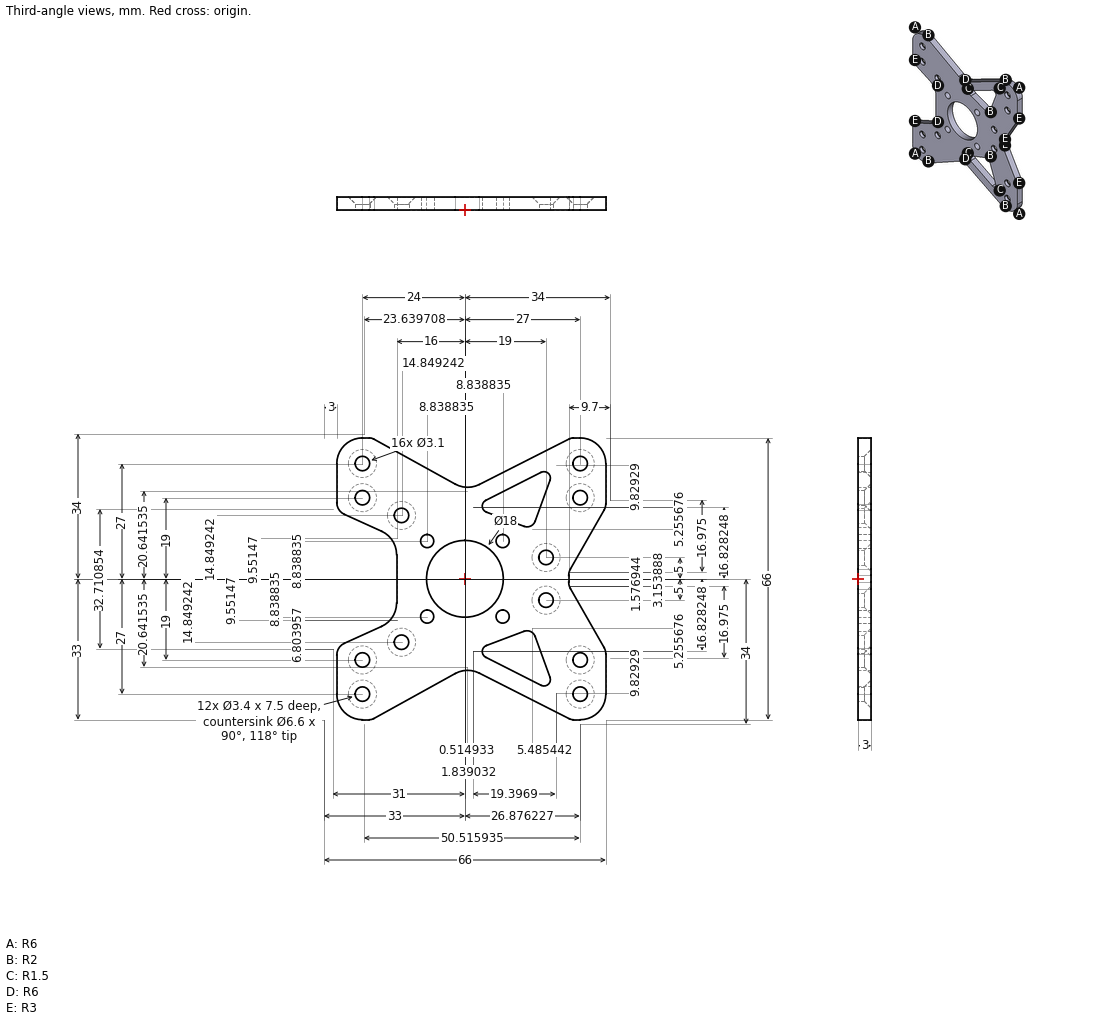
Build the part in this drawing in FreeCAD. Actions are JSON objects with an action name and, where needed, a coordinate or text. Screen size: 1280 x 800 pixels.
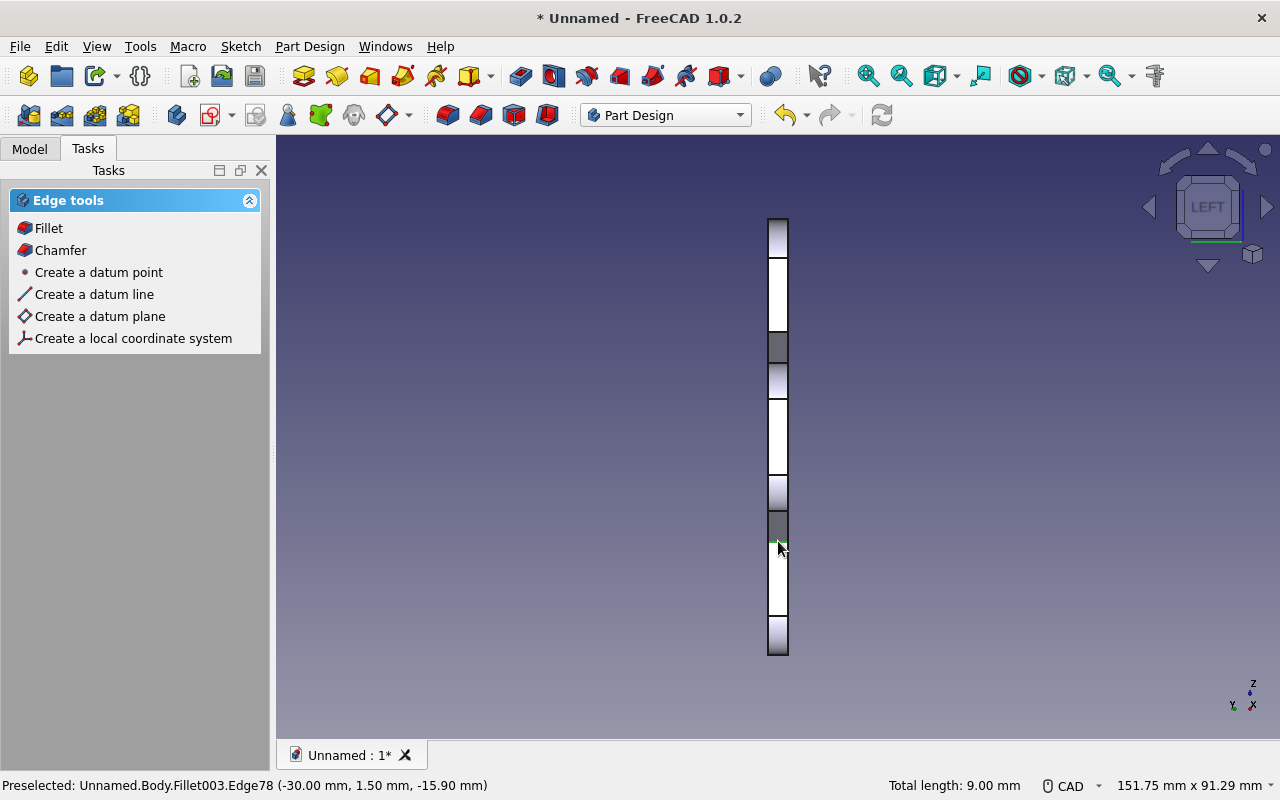
{"action": "left_click", "coordinate": [778, 331], "text": "ctrl"}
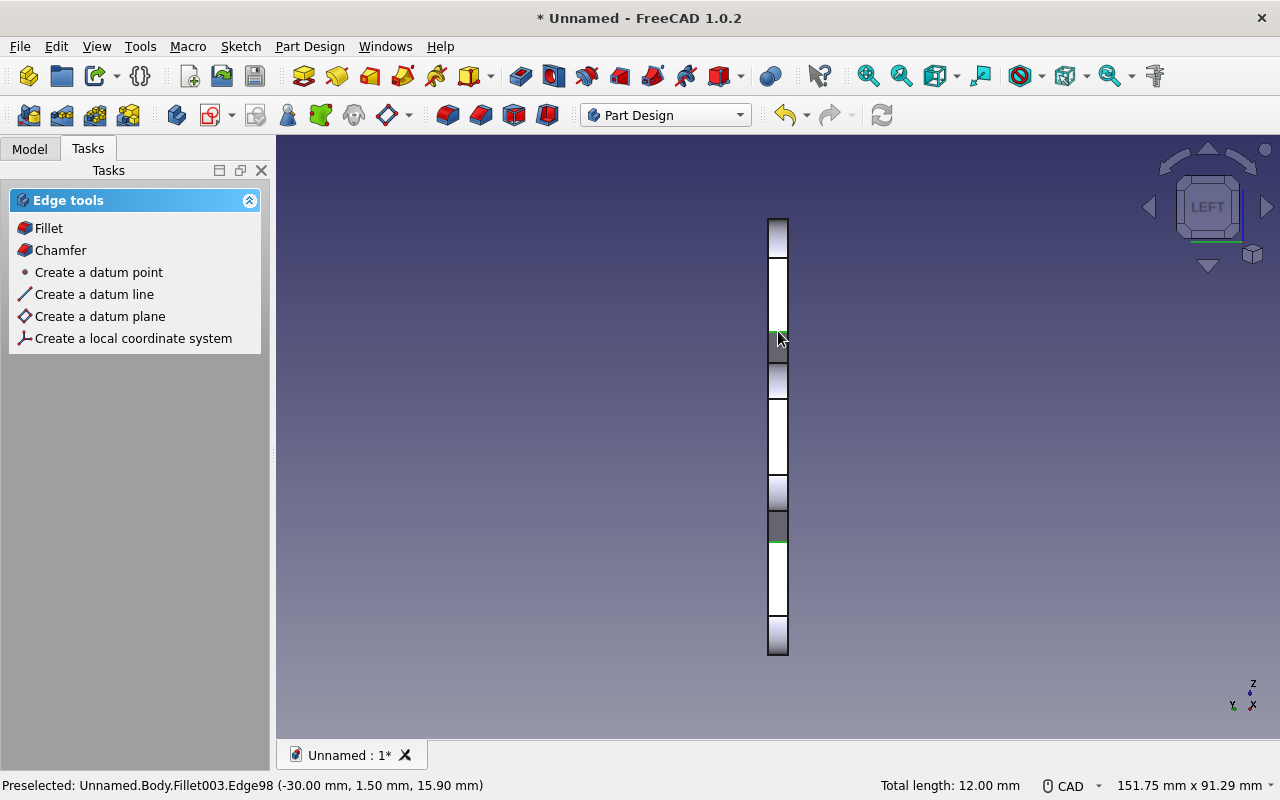
{"action": "scroll", "coordinate": [778, 446], "scroll_direction": "up", "scroll_amount": 4}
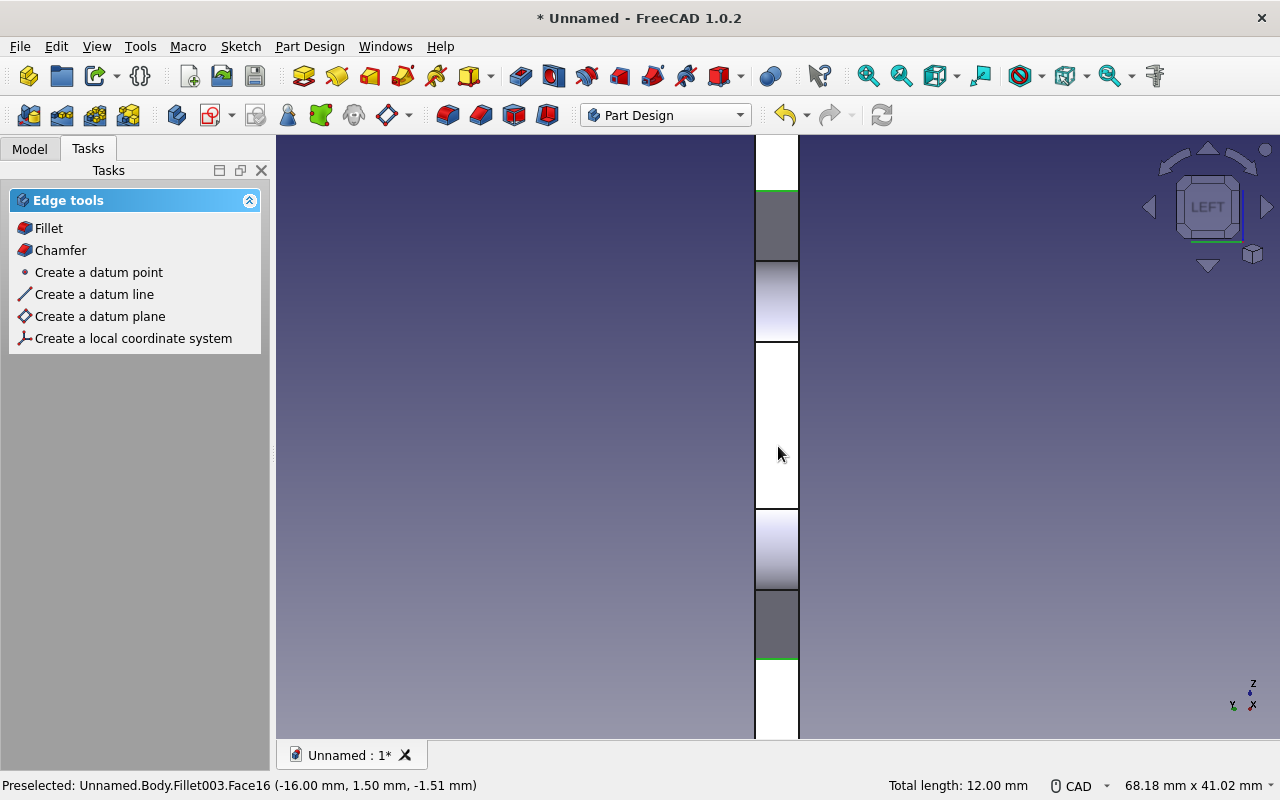
{"action": "key", "text": "v f"}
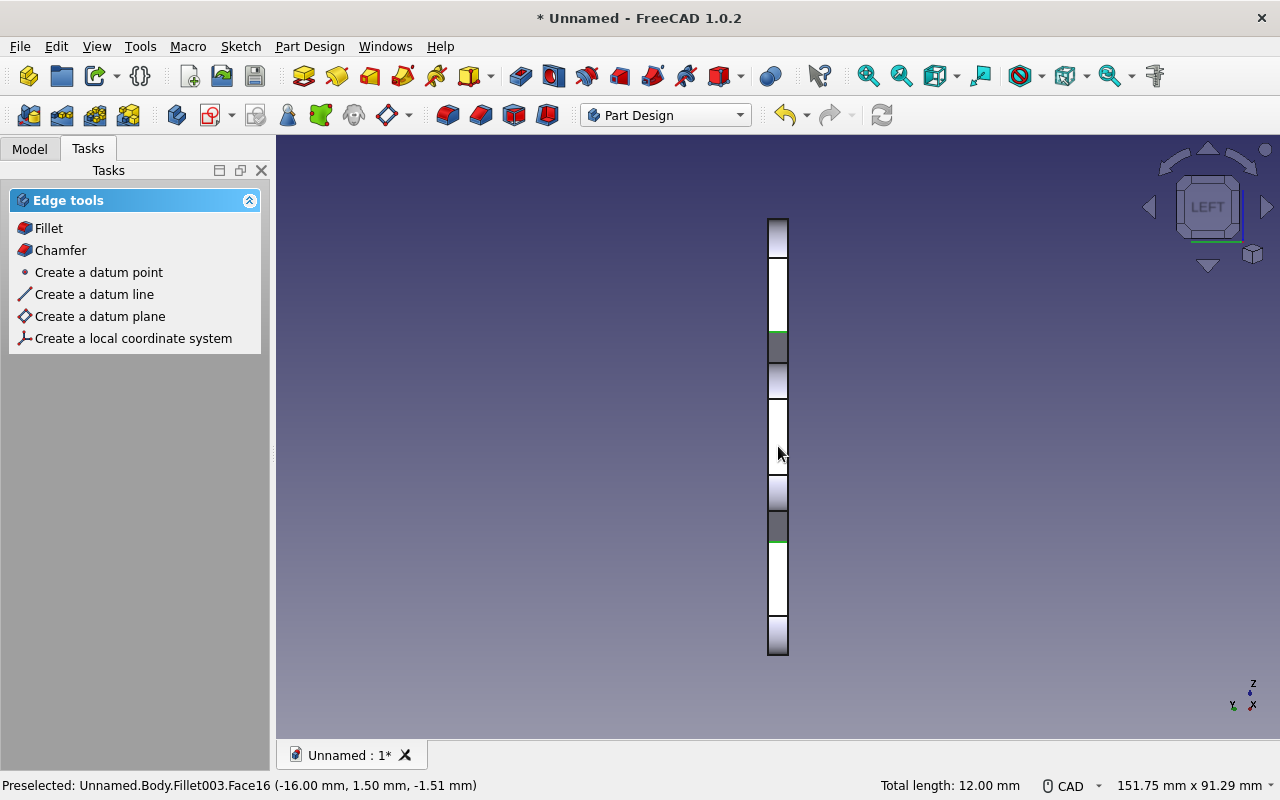
{"action": "key", "text": "v 3"}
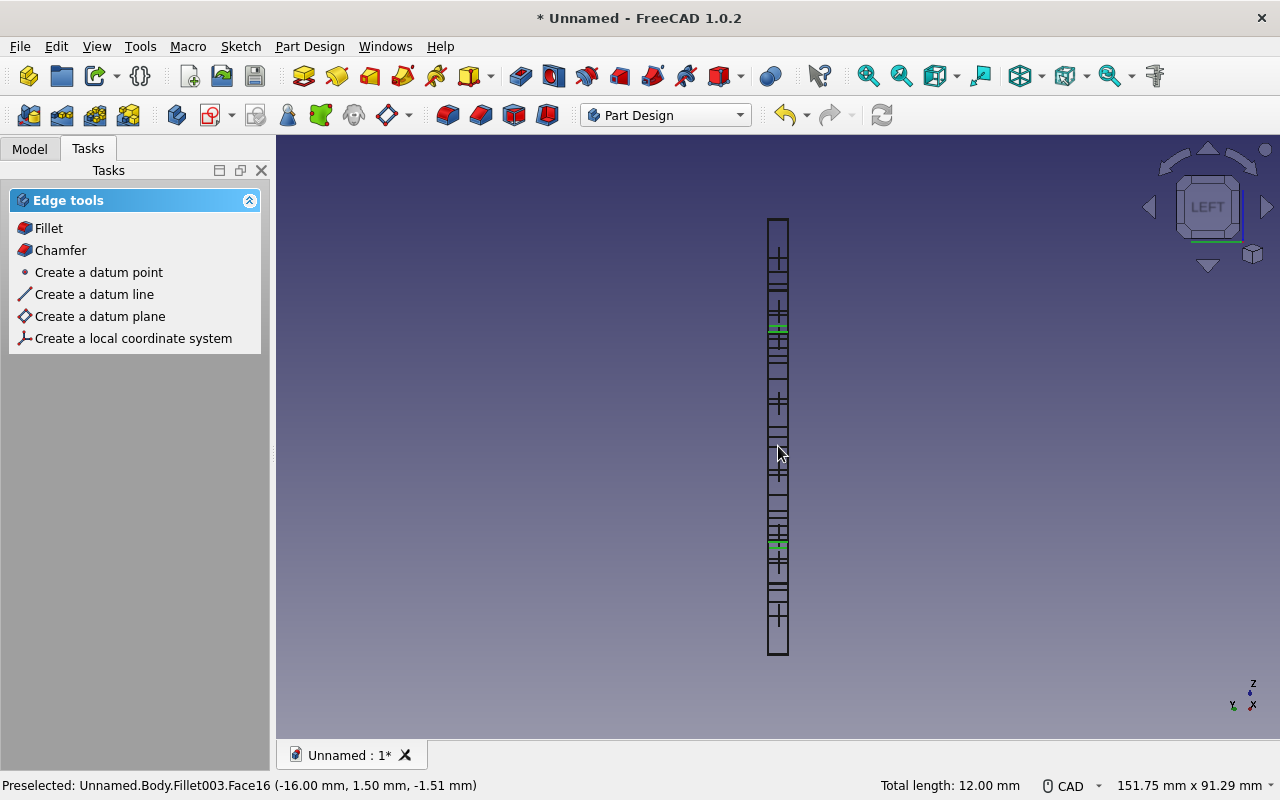
{"action": "key", "text": "0"}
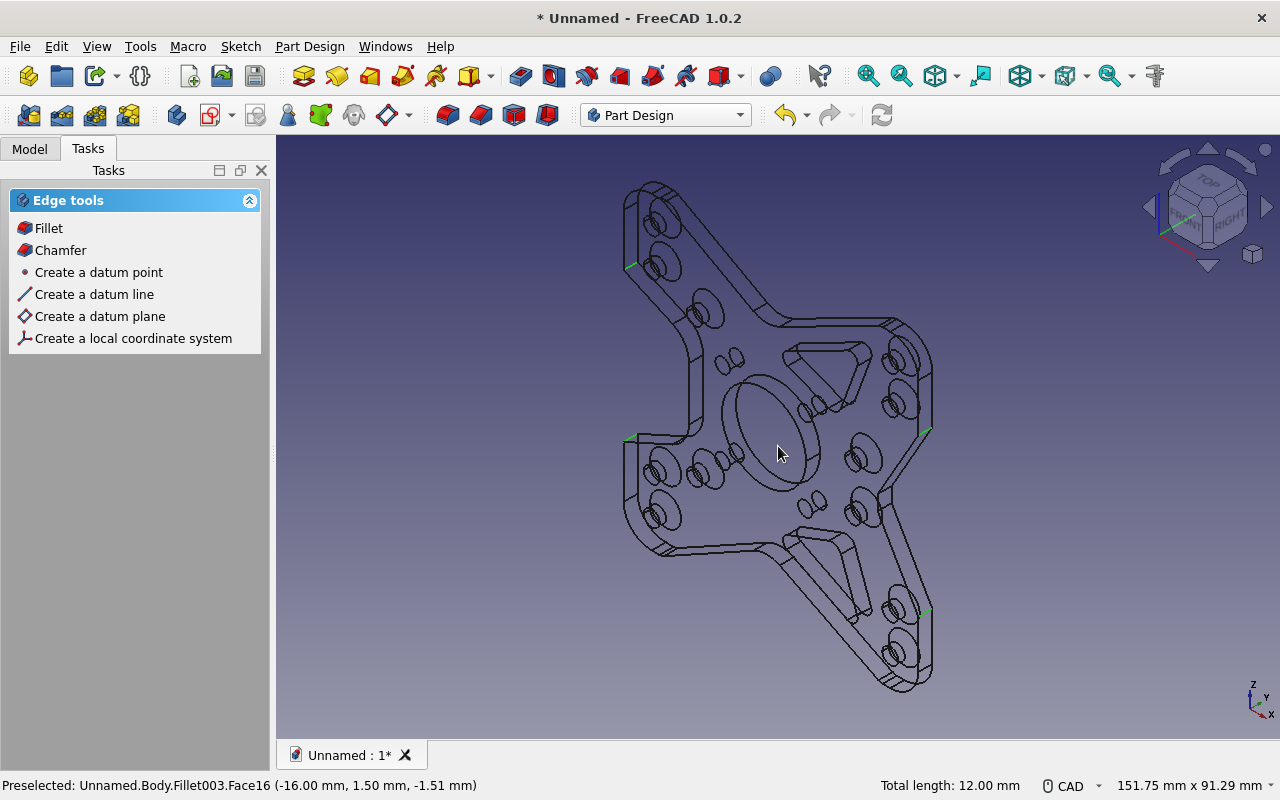
{"action": "left_click", "coordinate": [885, 506], "text": "ctrl"}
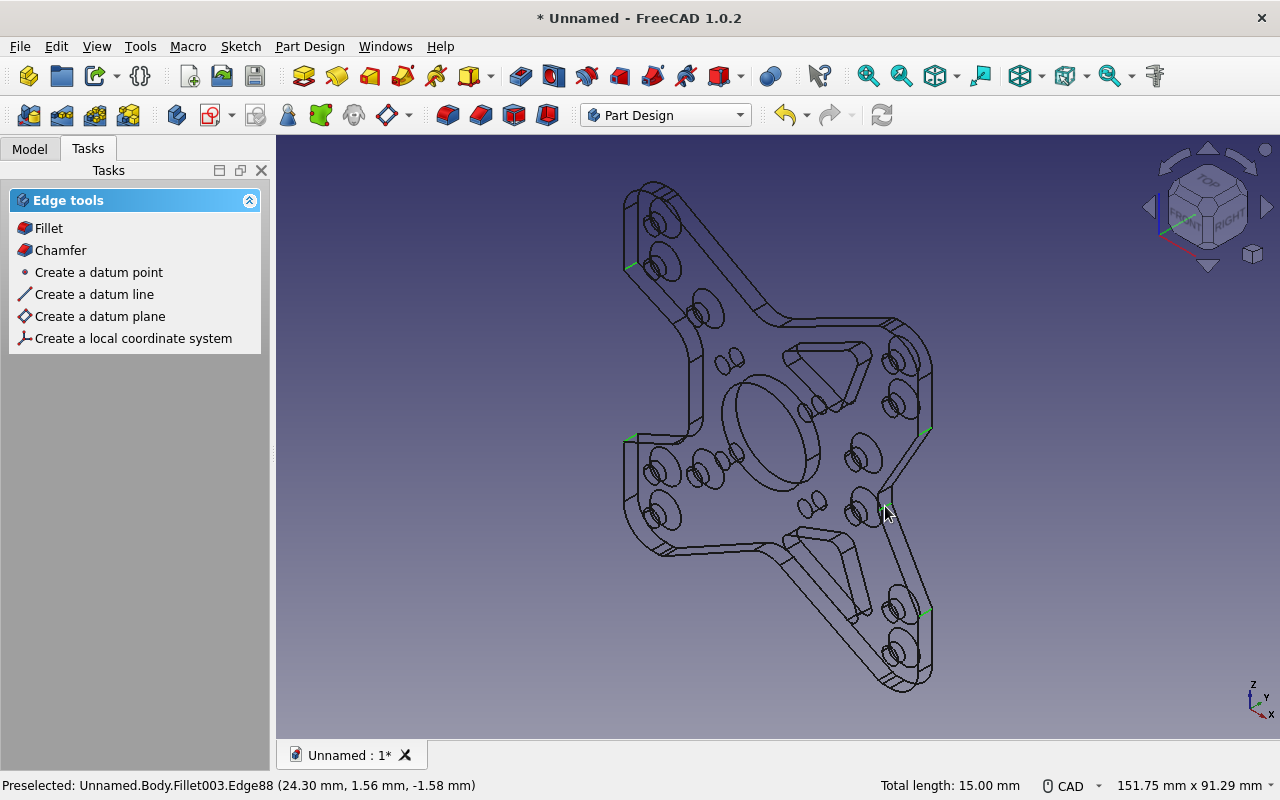
{"action": "scroll", "coordinate": [885, 489], "scroll_direction": "up", "scroll_amount": 6}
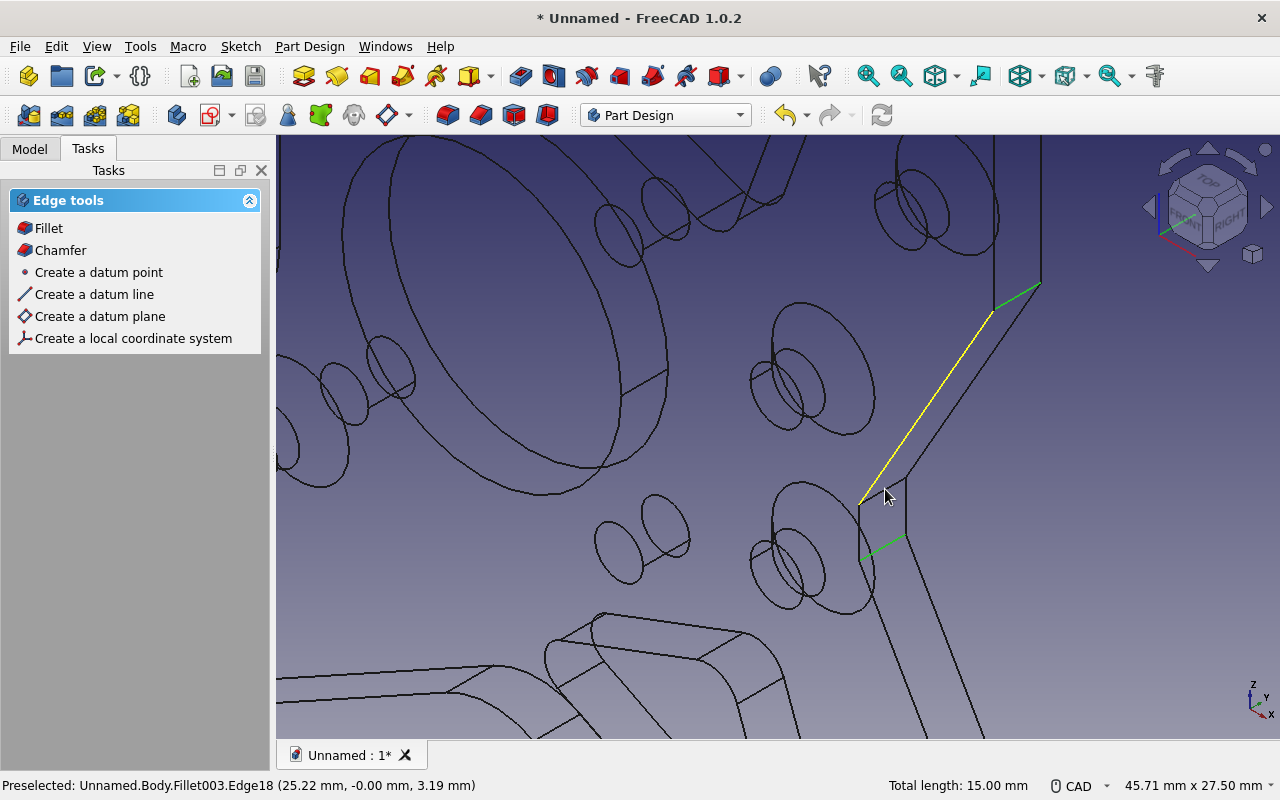
{"action": "left_click", "coordinate": [882, 490], "text": "ctrl"}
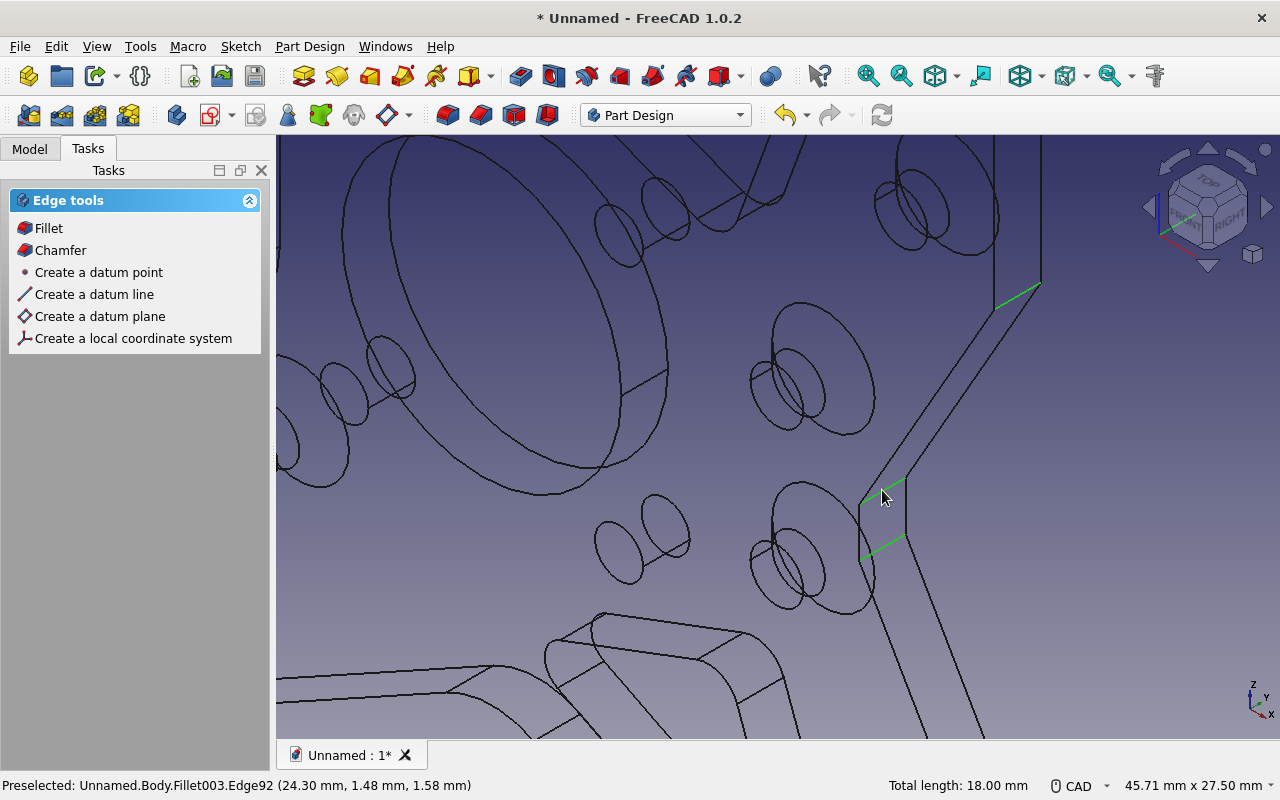
{"action": "key", "text": "v 1"}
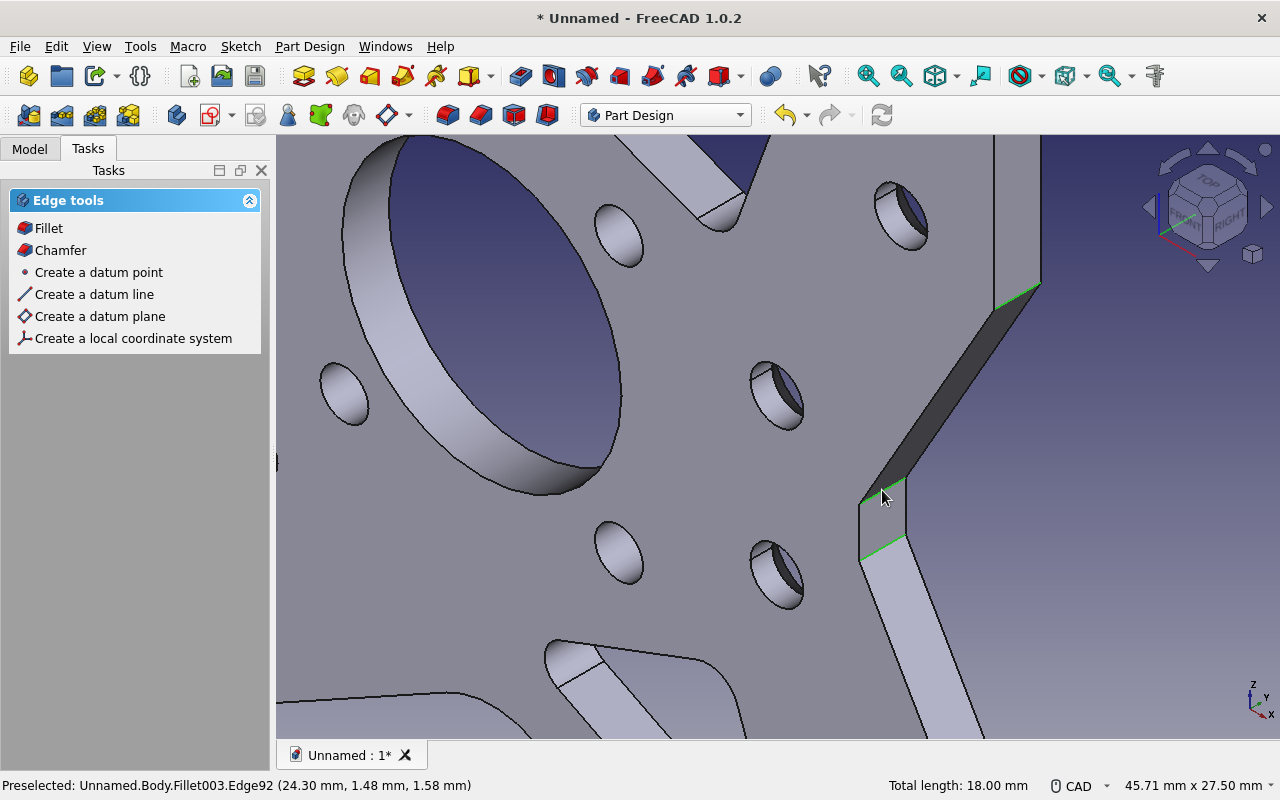
{"action": "left_click", "coordinate": [448, 116]}